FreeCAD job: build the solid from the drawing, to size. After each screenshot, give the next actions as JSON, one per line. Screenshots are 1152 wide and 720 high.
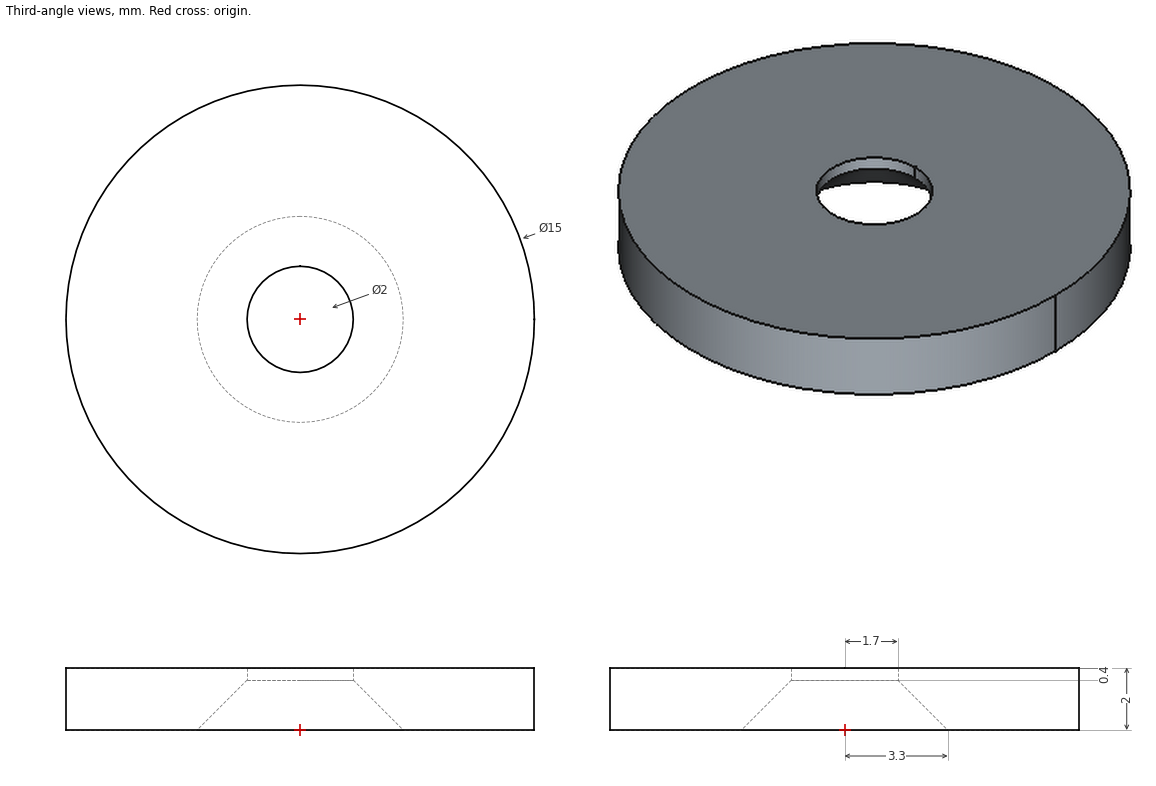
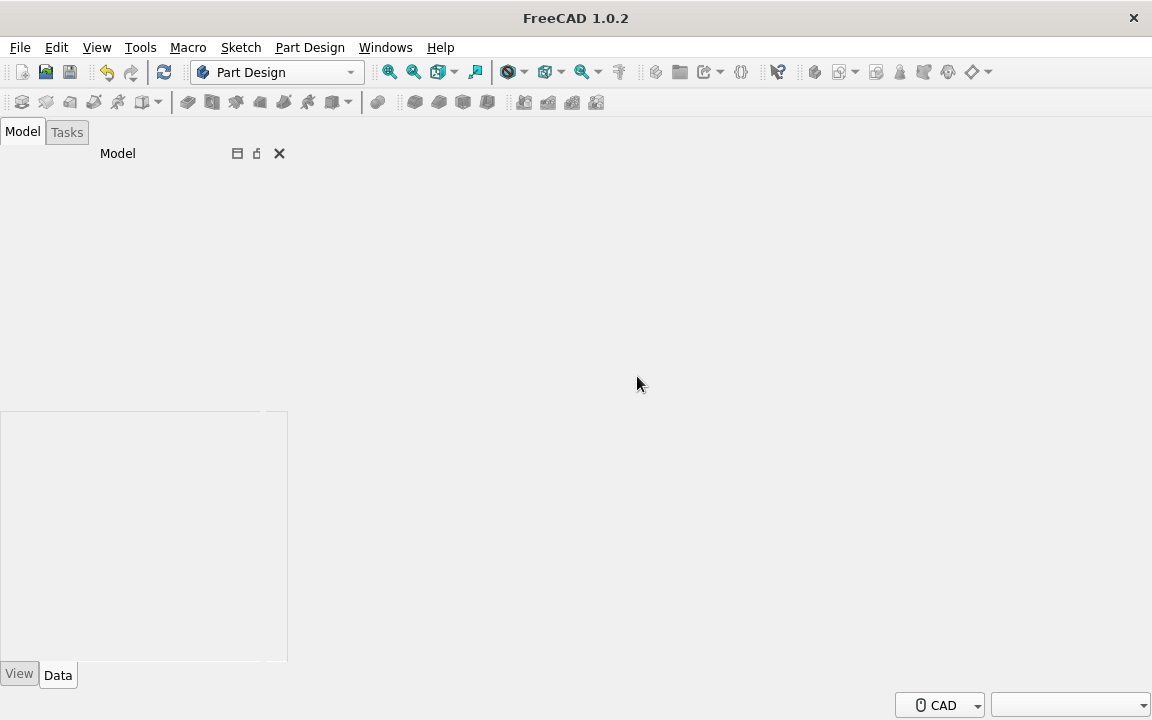
{"action": "left_click", "coordinate": [22, 72]}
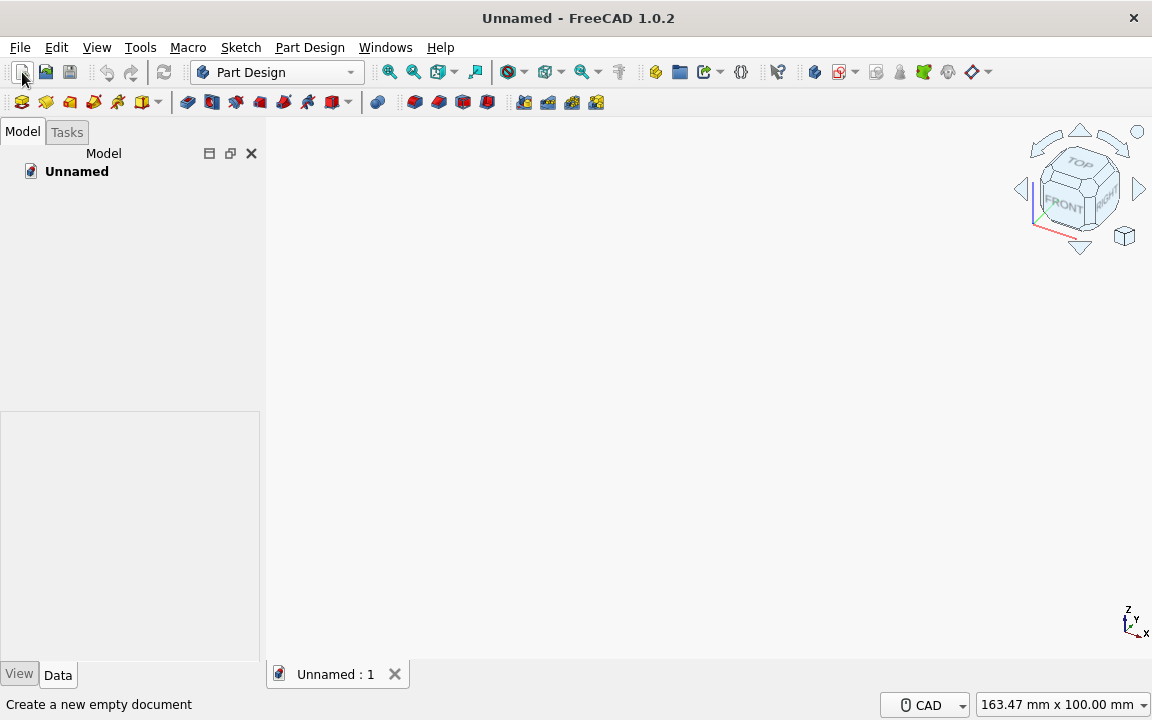
{"action": "left_click", "coordinate": [840, 72]}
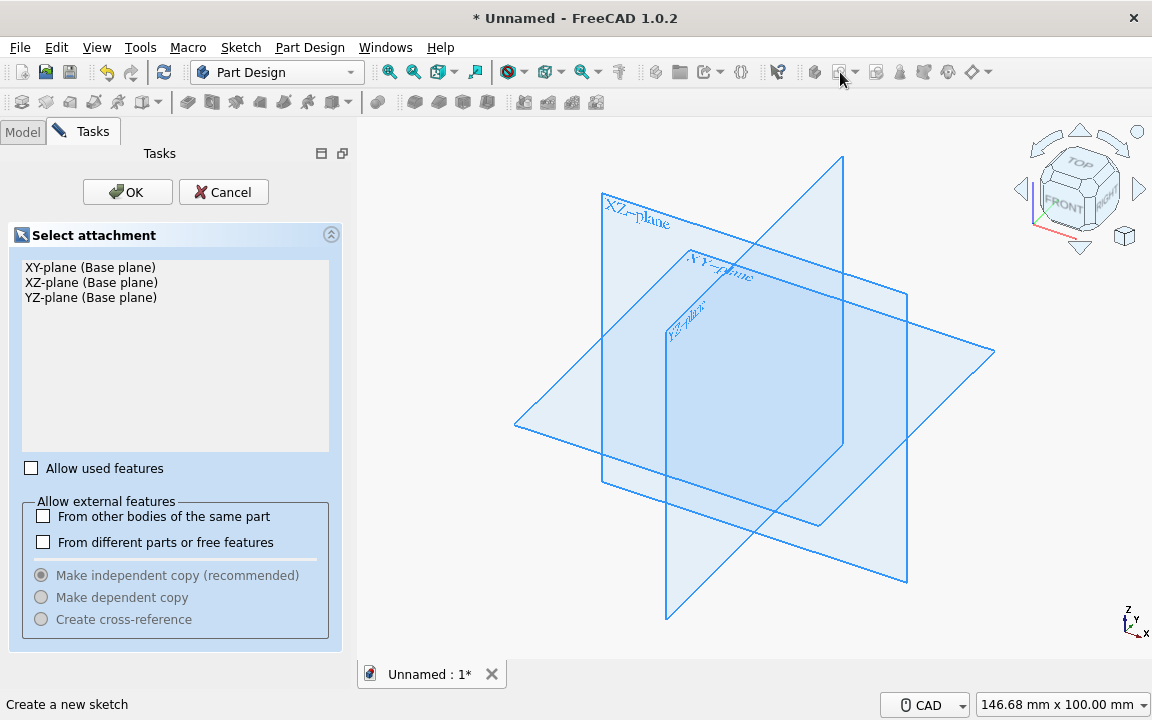
{"action": "left_click", "coordinate": [82, 268]}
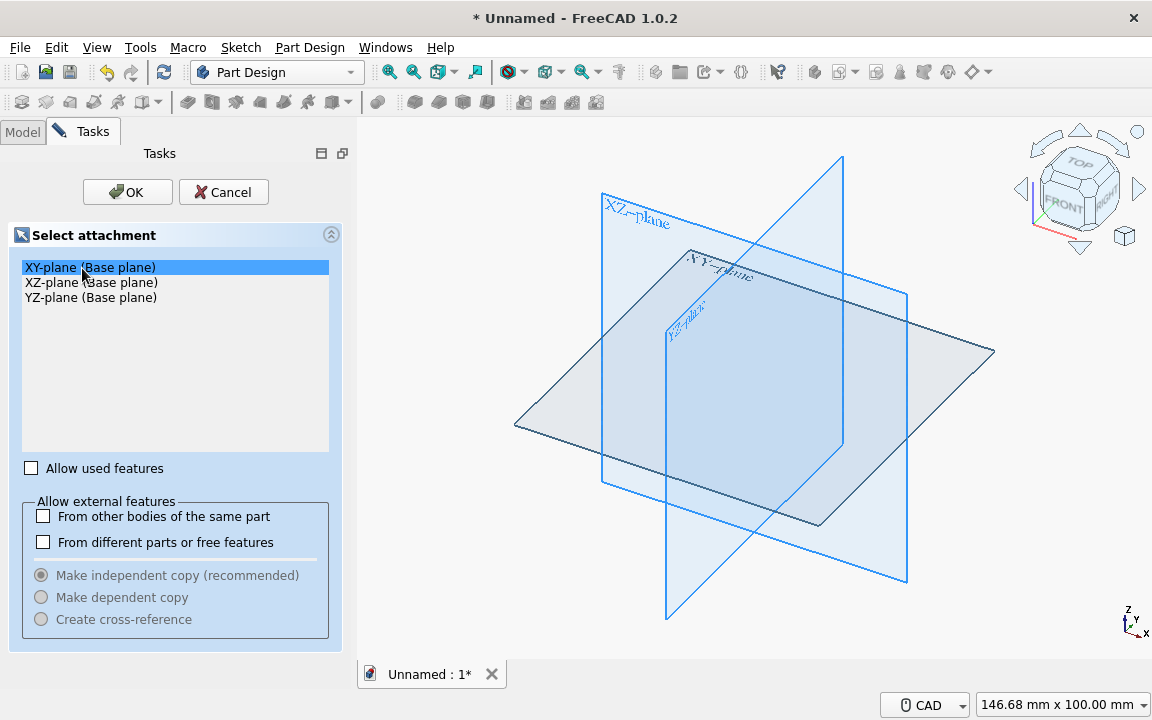
{"action": "left_click", "coordinate": [128, 192]}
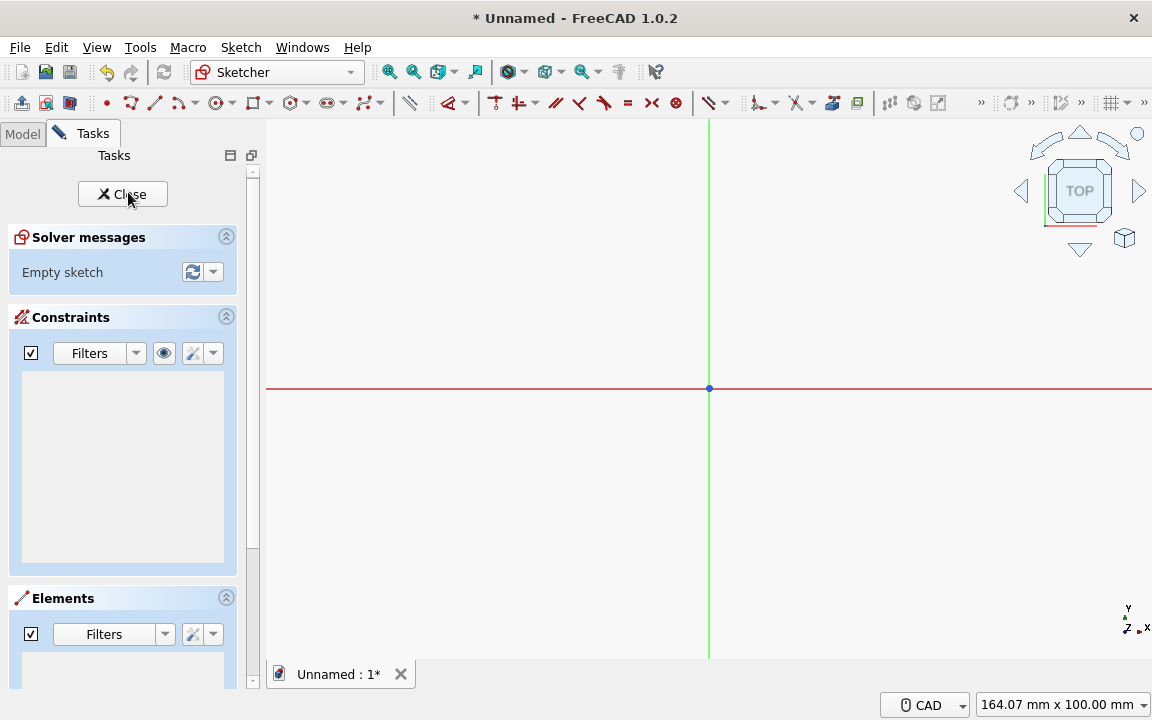
{"action": "scroll", "coordinate": [731, 389], "scroll_direction": "up", "scroll_amount": 7}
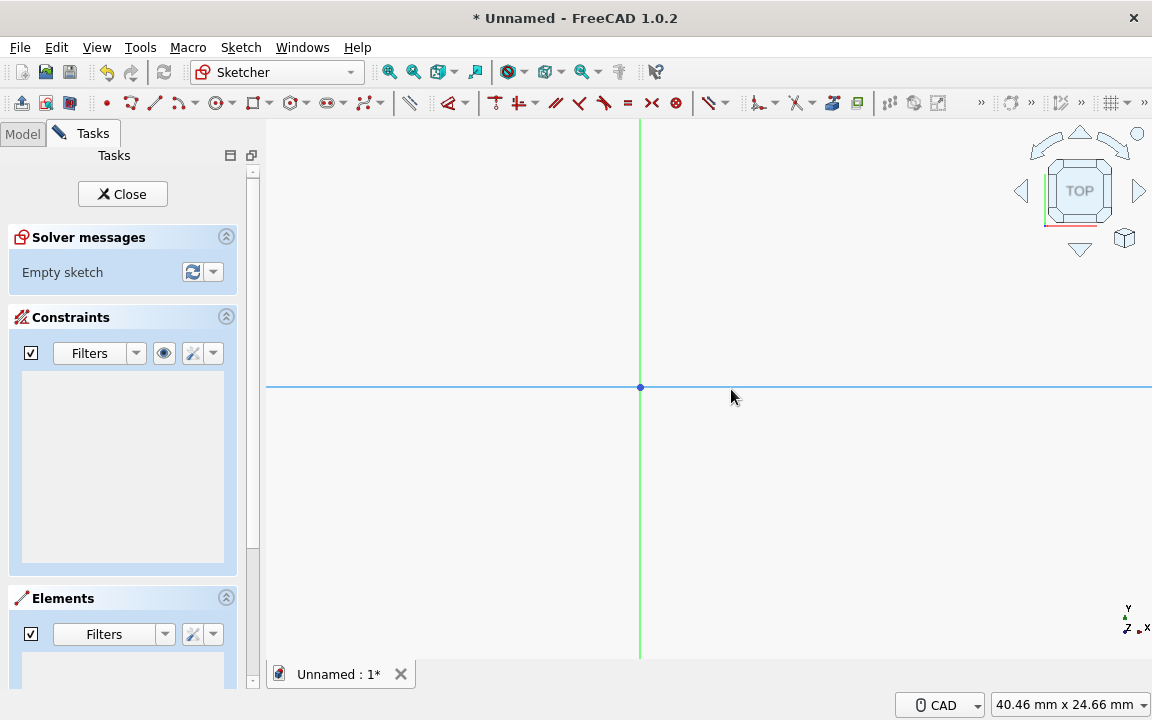
{"action": "left_click", "coordinate": [216, 104]}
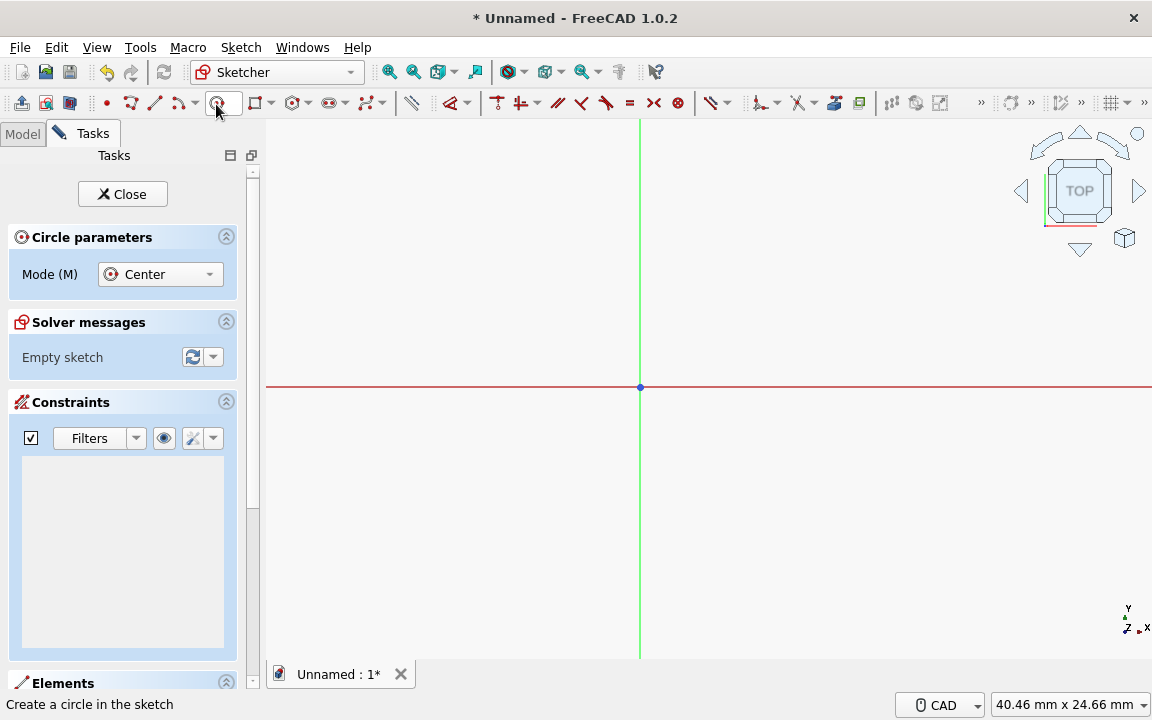
{"action": "left_click", "coordinate": [640, 387]}
{"action": "mouse_move", "coordinate": [756, 271]}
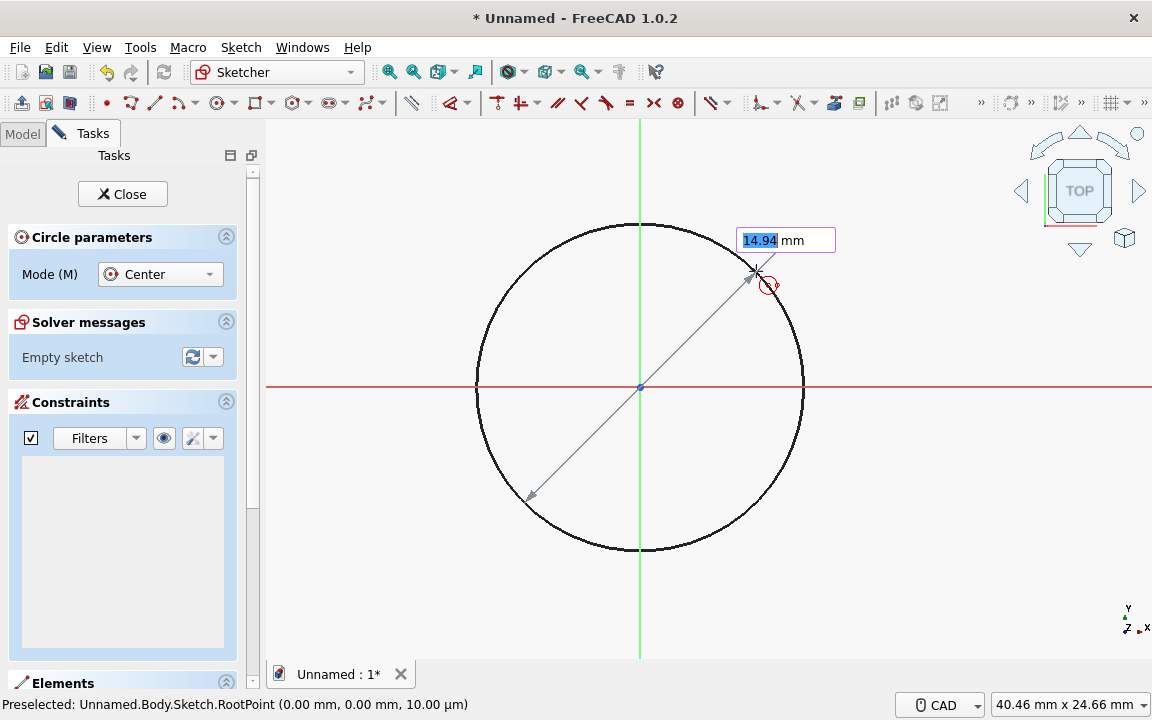
{"action": "type", "text": "15"}
{"action": "key", "text": "Return"}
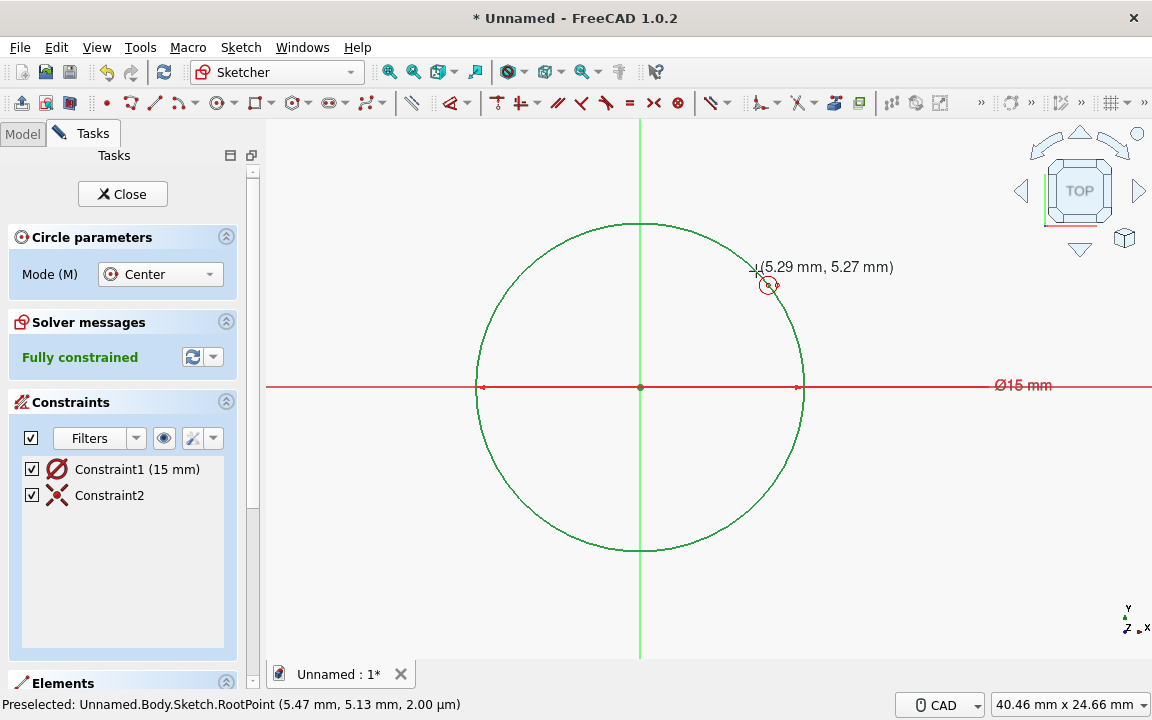
{"action": "left_click", "coordinate": [640, 387]}
{"action": "mouse_move", "coordinate": [656, 372]}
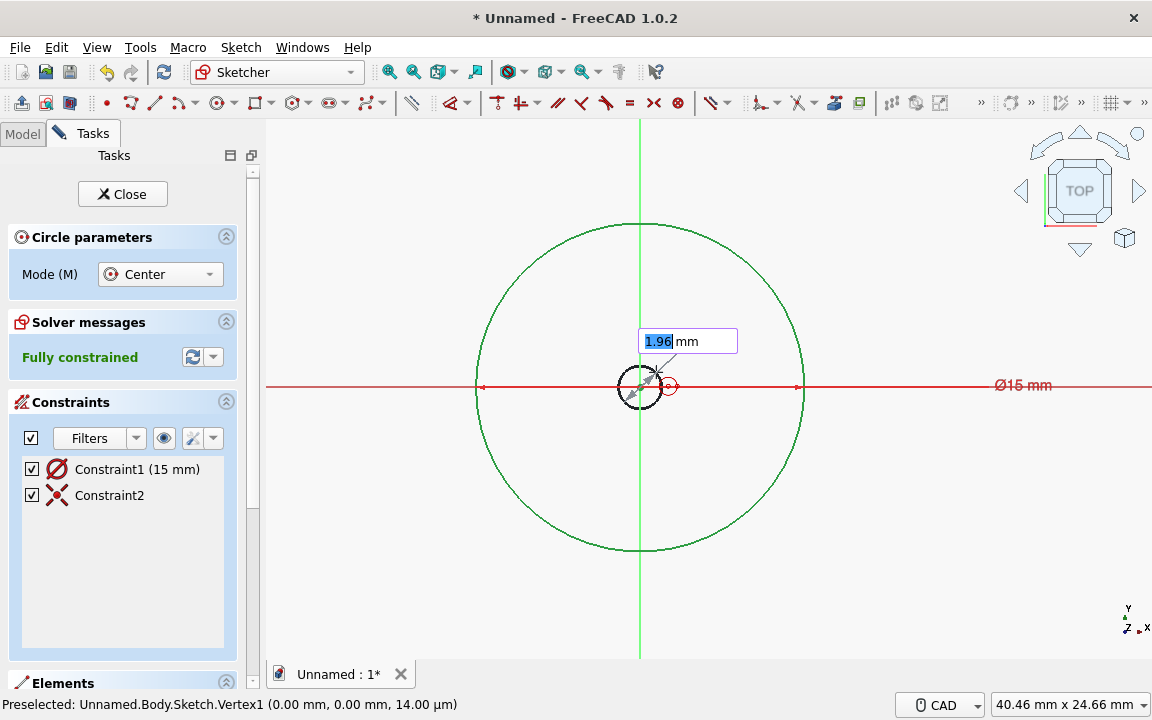
{"action": "type", "text": "2"}
{"action": "key", "text": "Return"}
{"action": "key", "text": "Escape"}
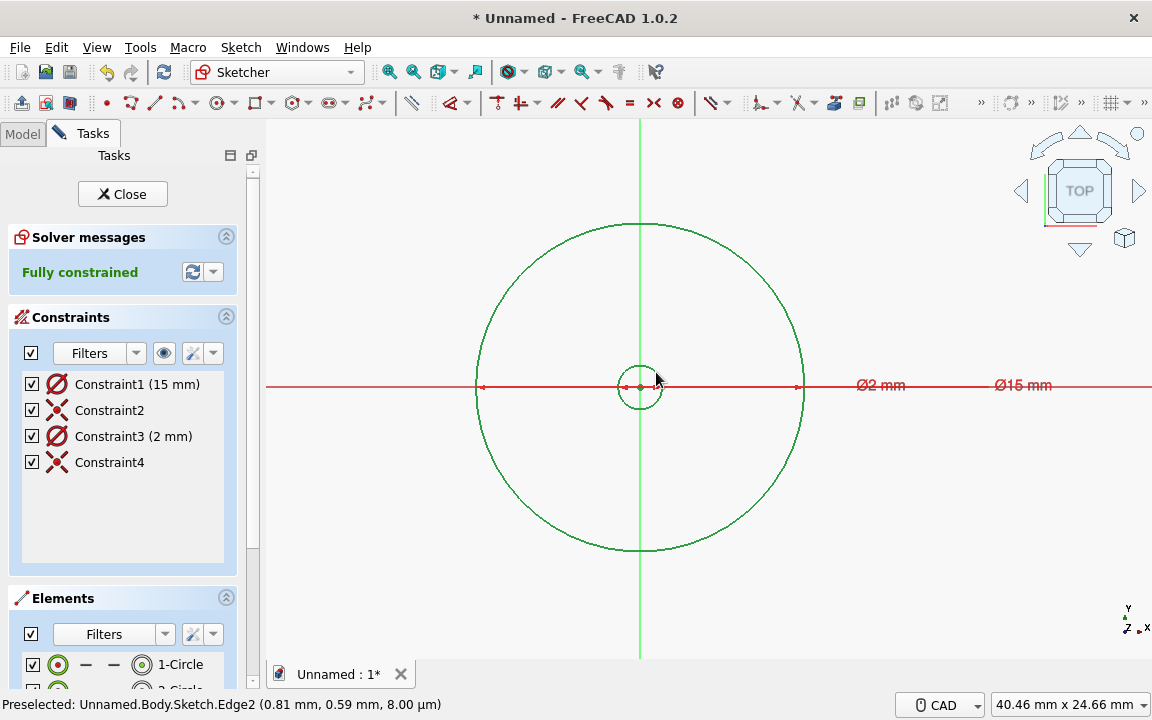
{"action": "left_click", "coordinate": [123, 194]}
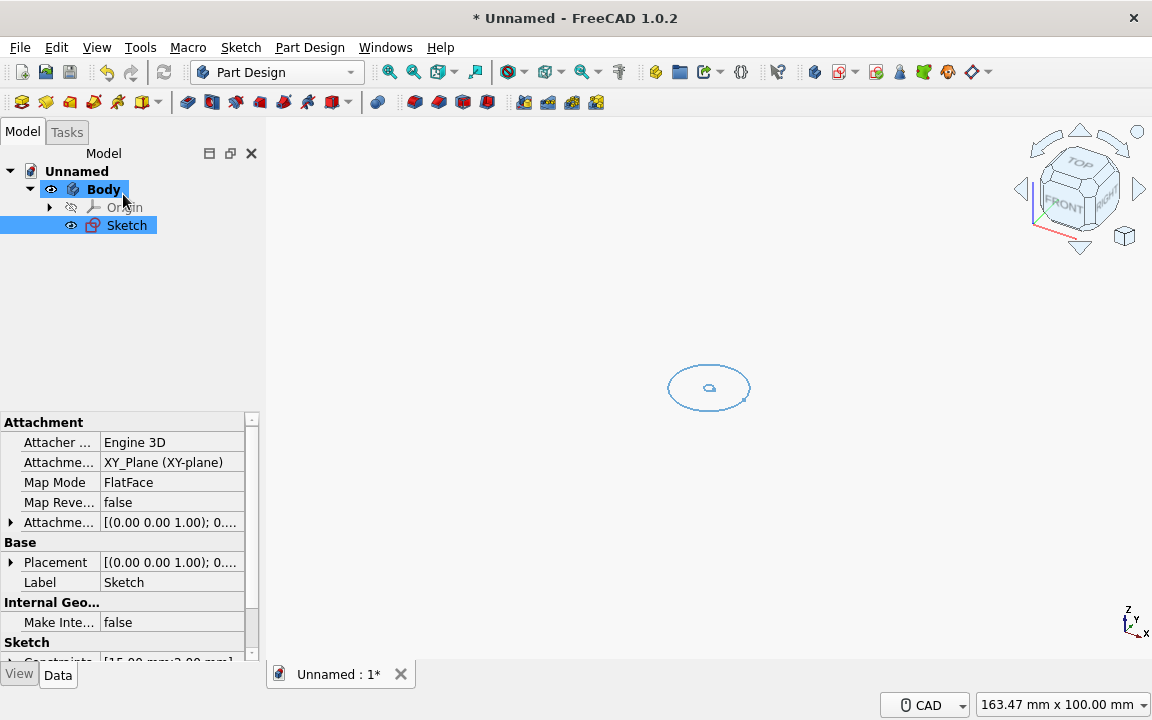
{"action": "left_click", "coordinate": [22, 102]}